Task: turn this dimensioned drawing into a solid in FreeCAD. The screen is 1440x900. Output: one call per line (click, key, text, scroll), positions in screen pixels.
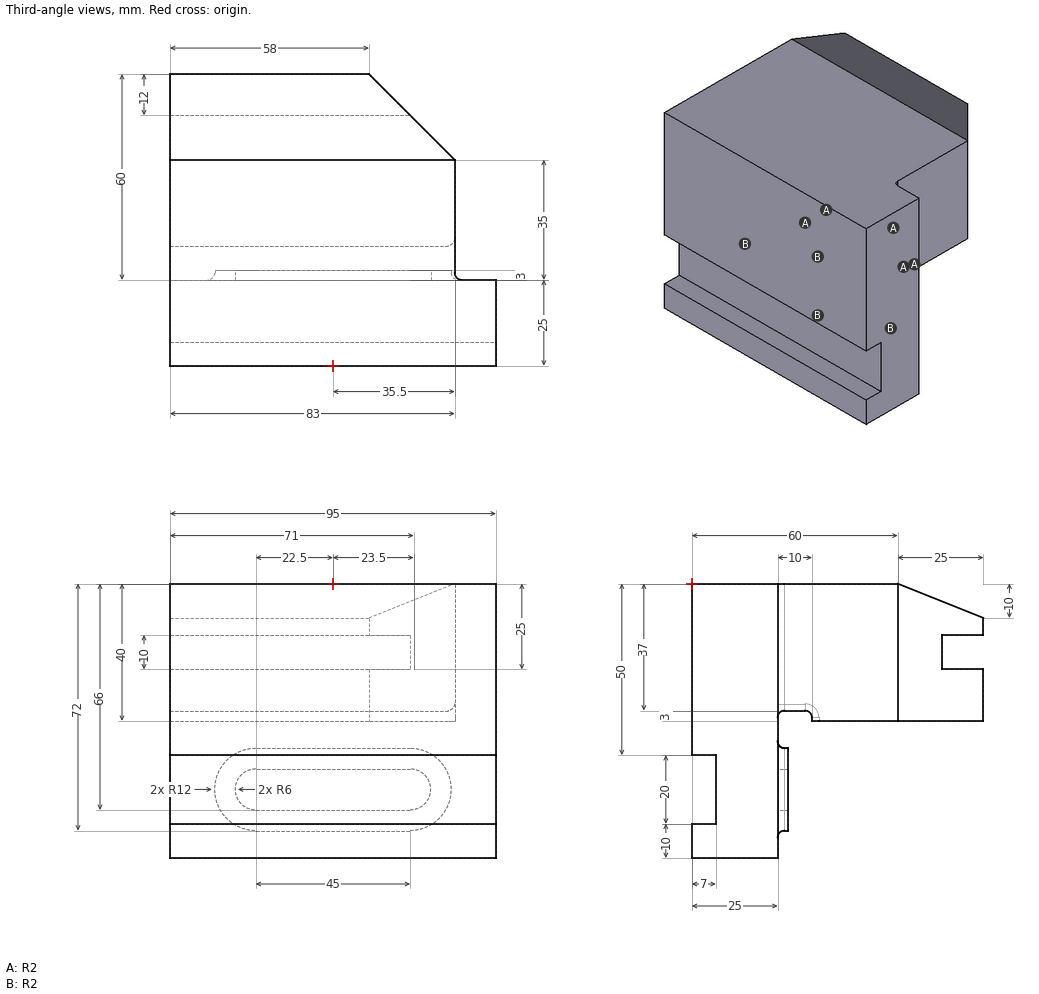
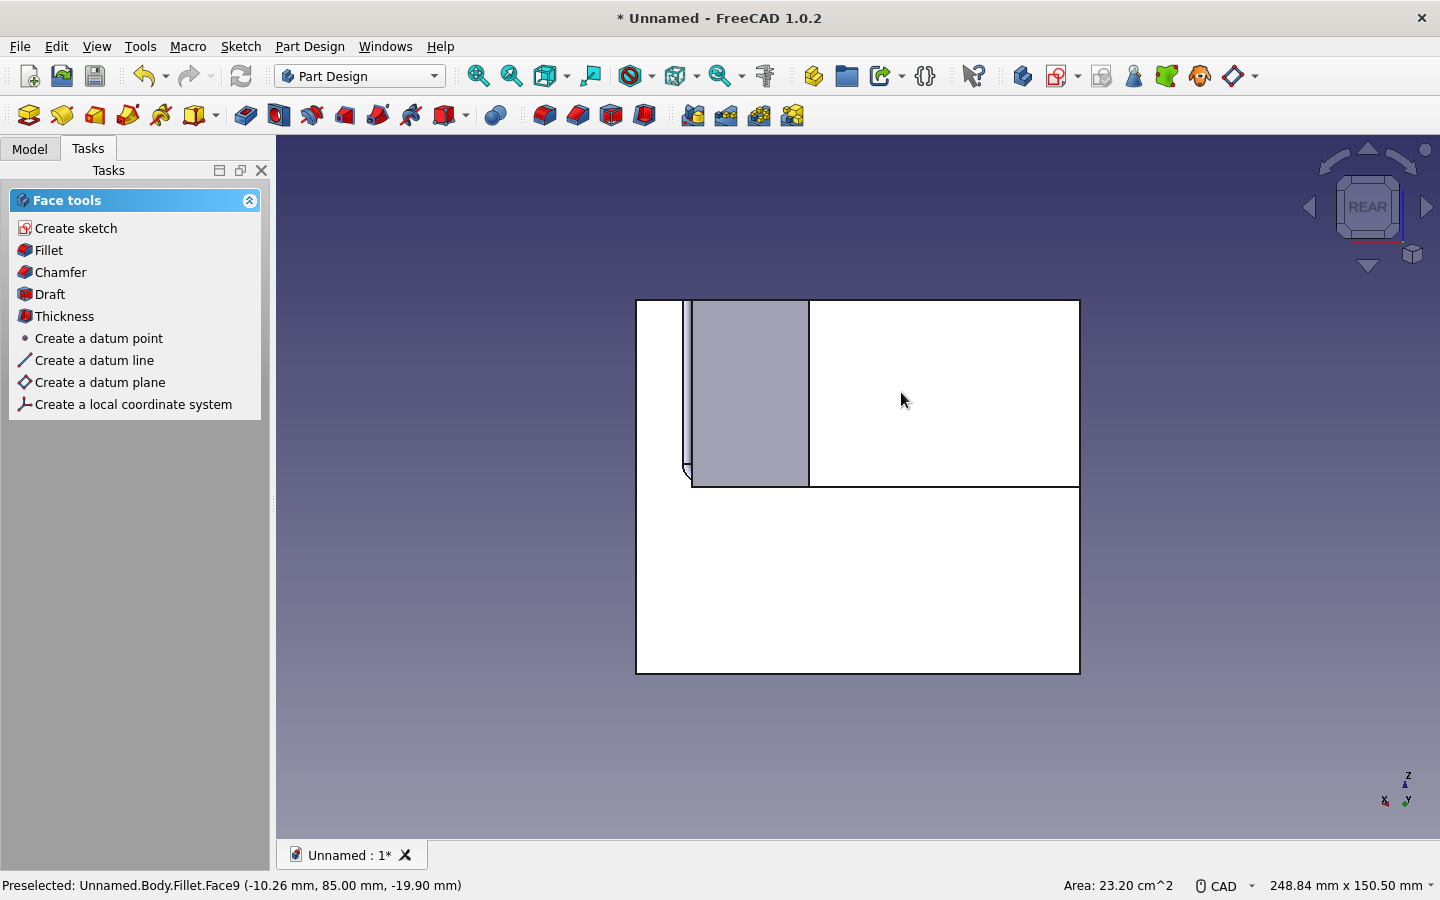
click(1056, 76)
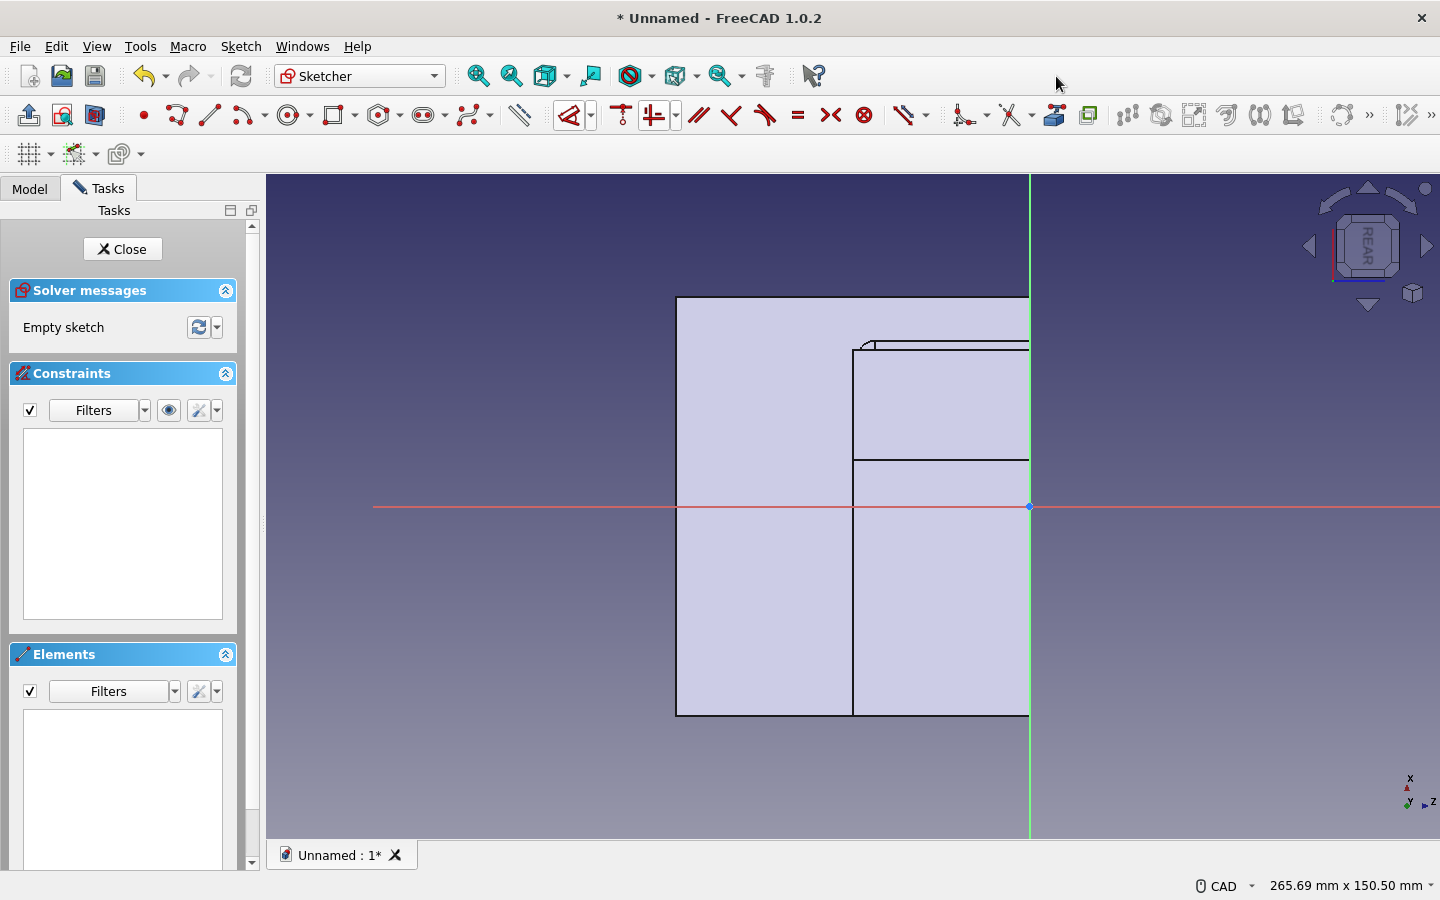
scroll(1275, 667, up, 2)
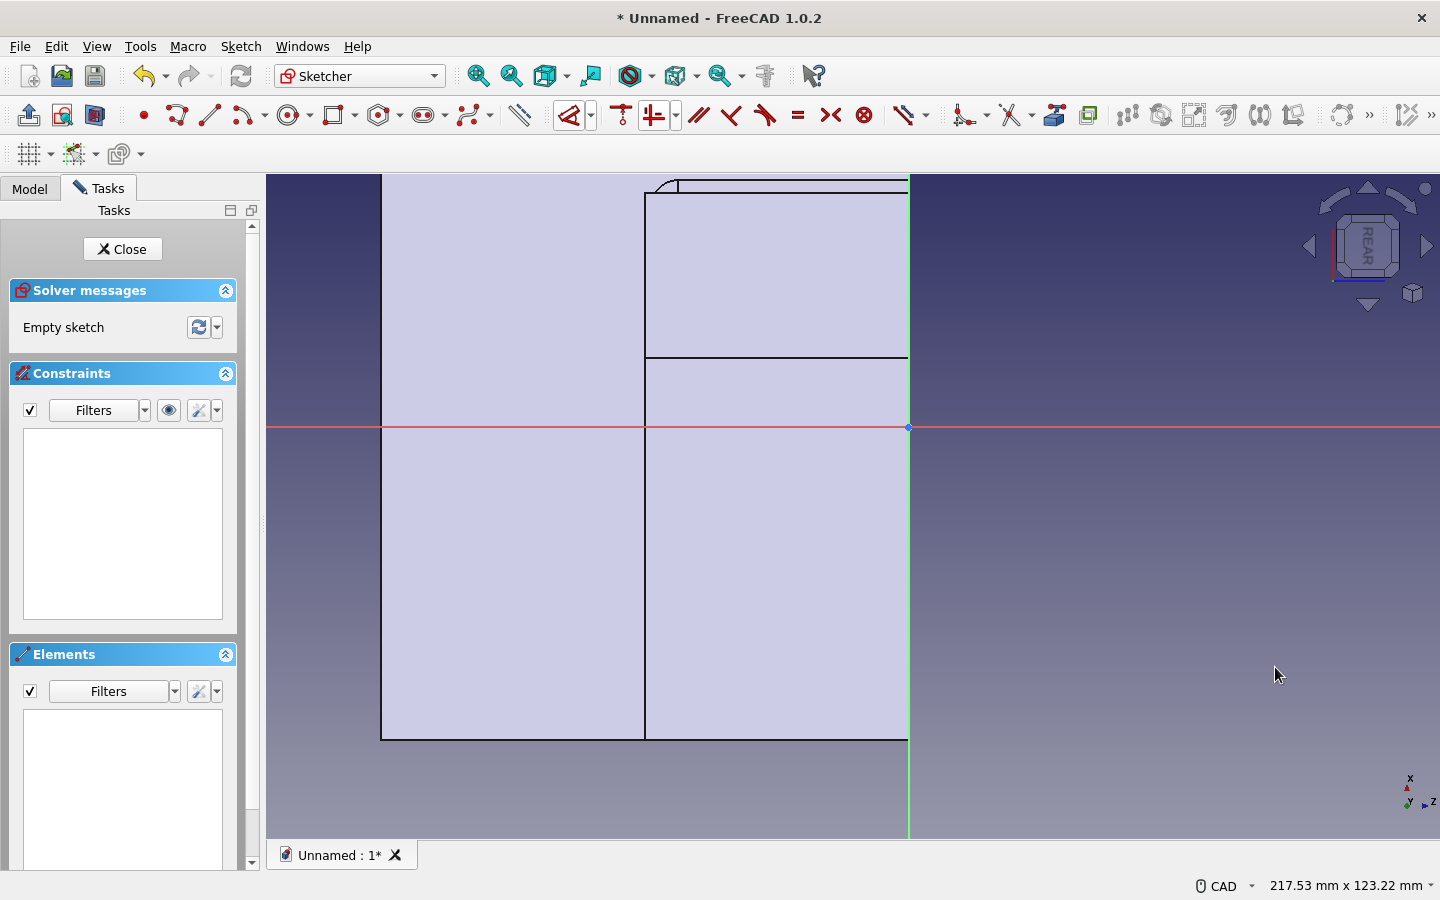
click(332, 116)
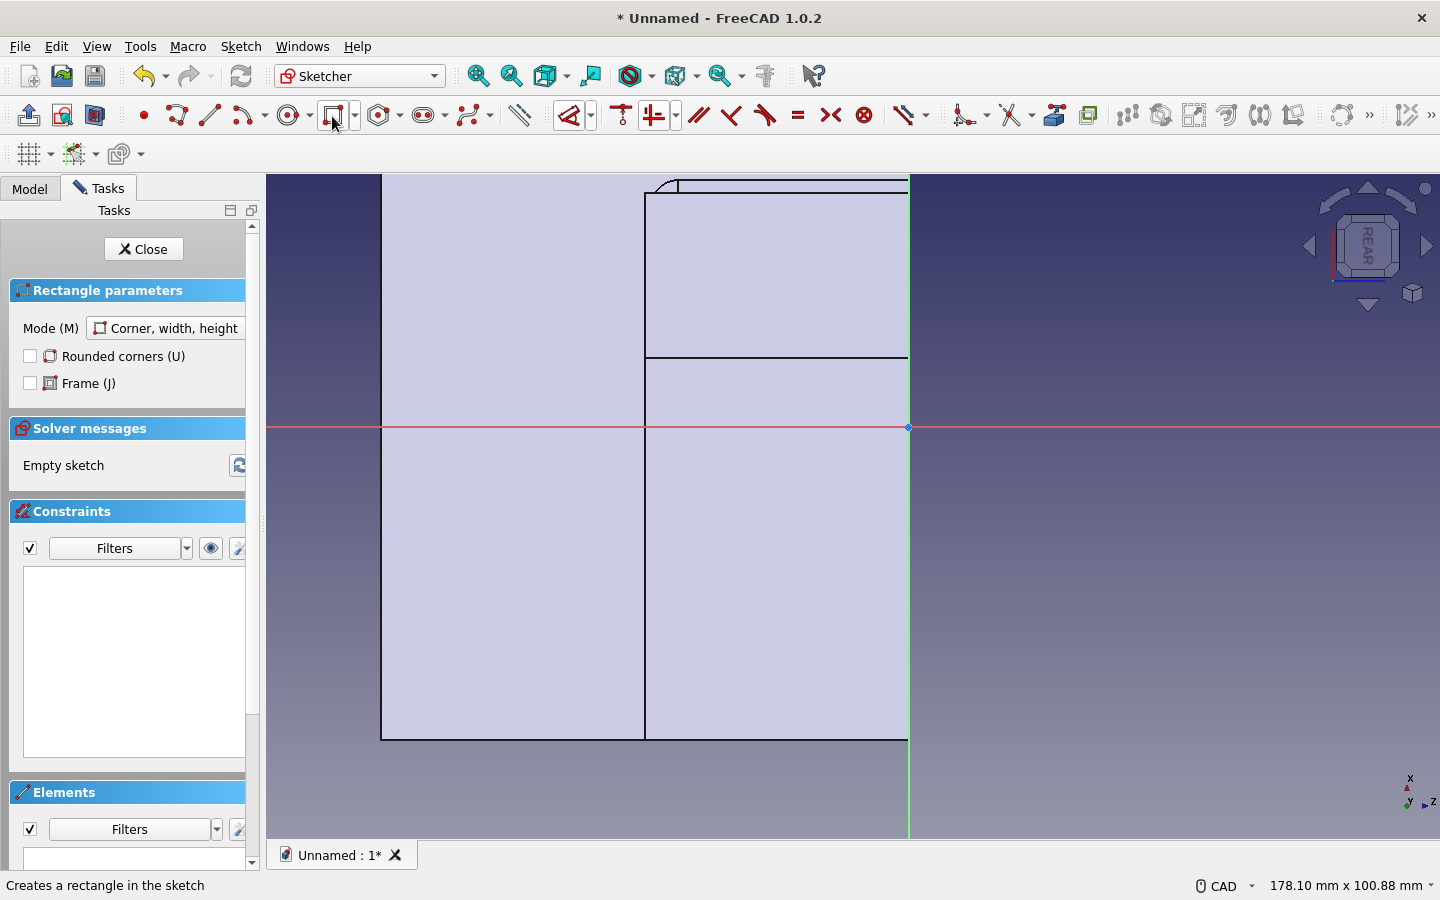
click(744, 272)
click(810, 740)
key(Escape)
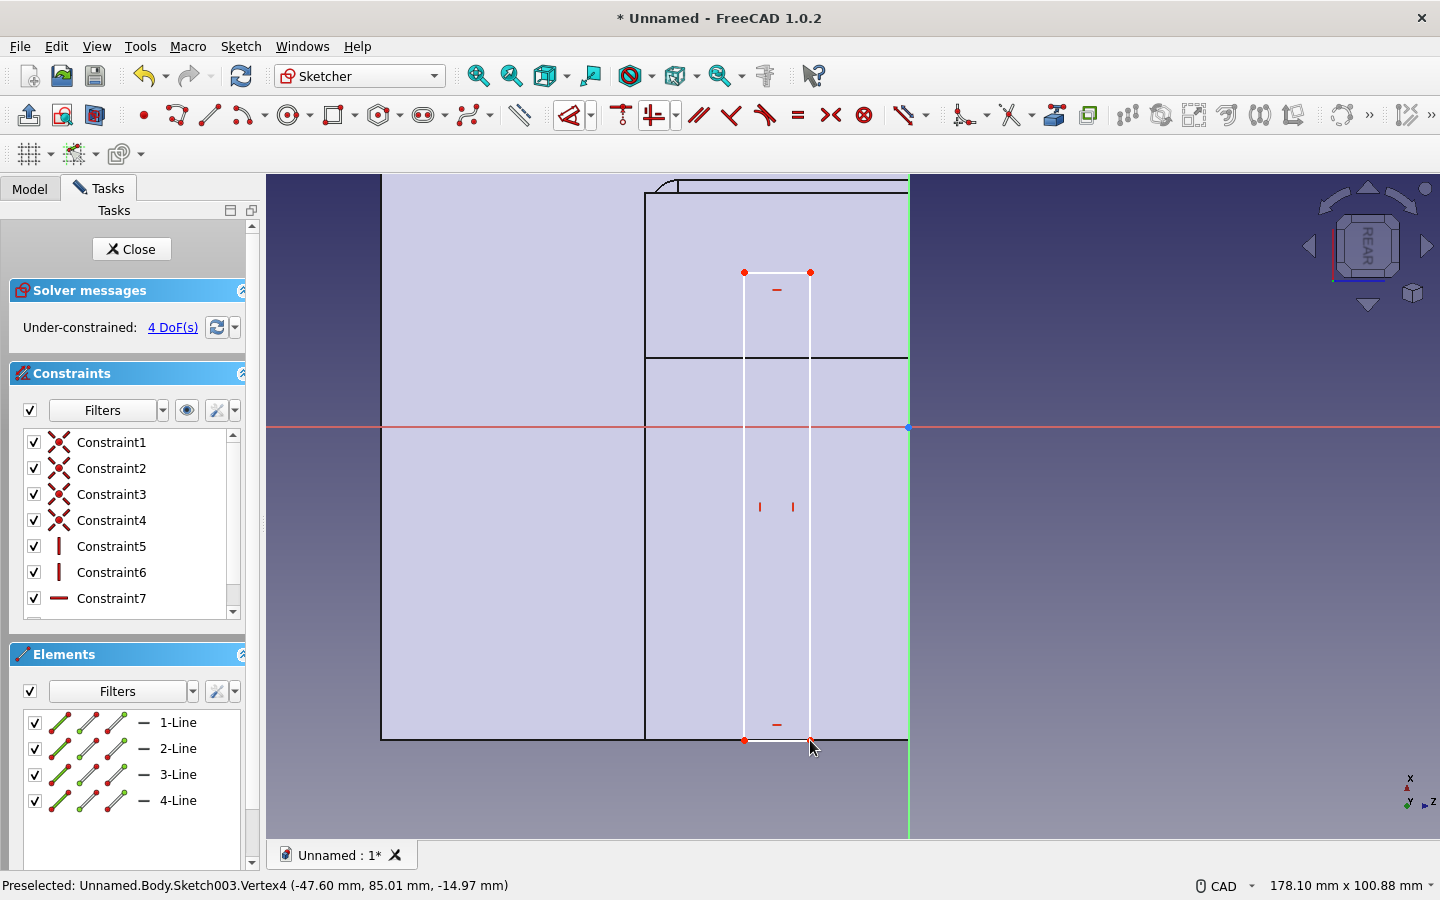
click(744, 413)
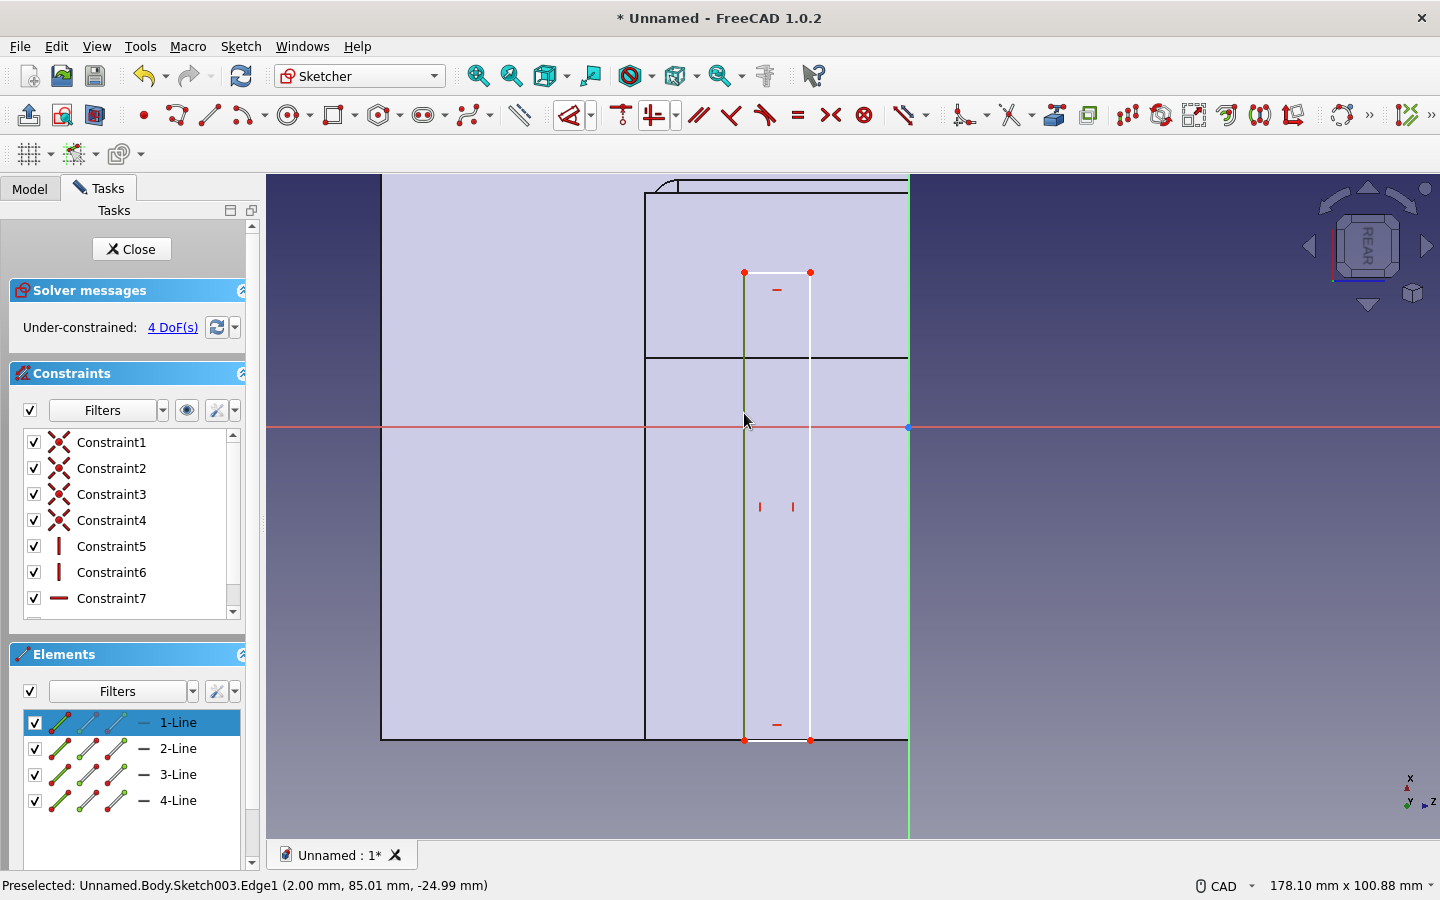
key(i)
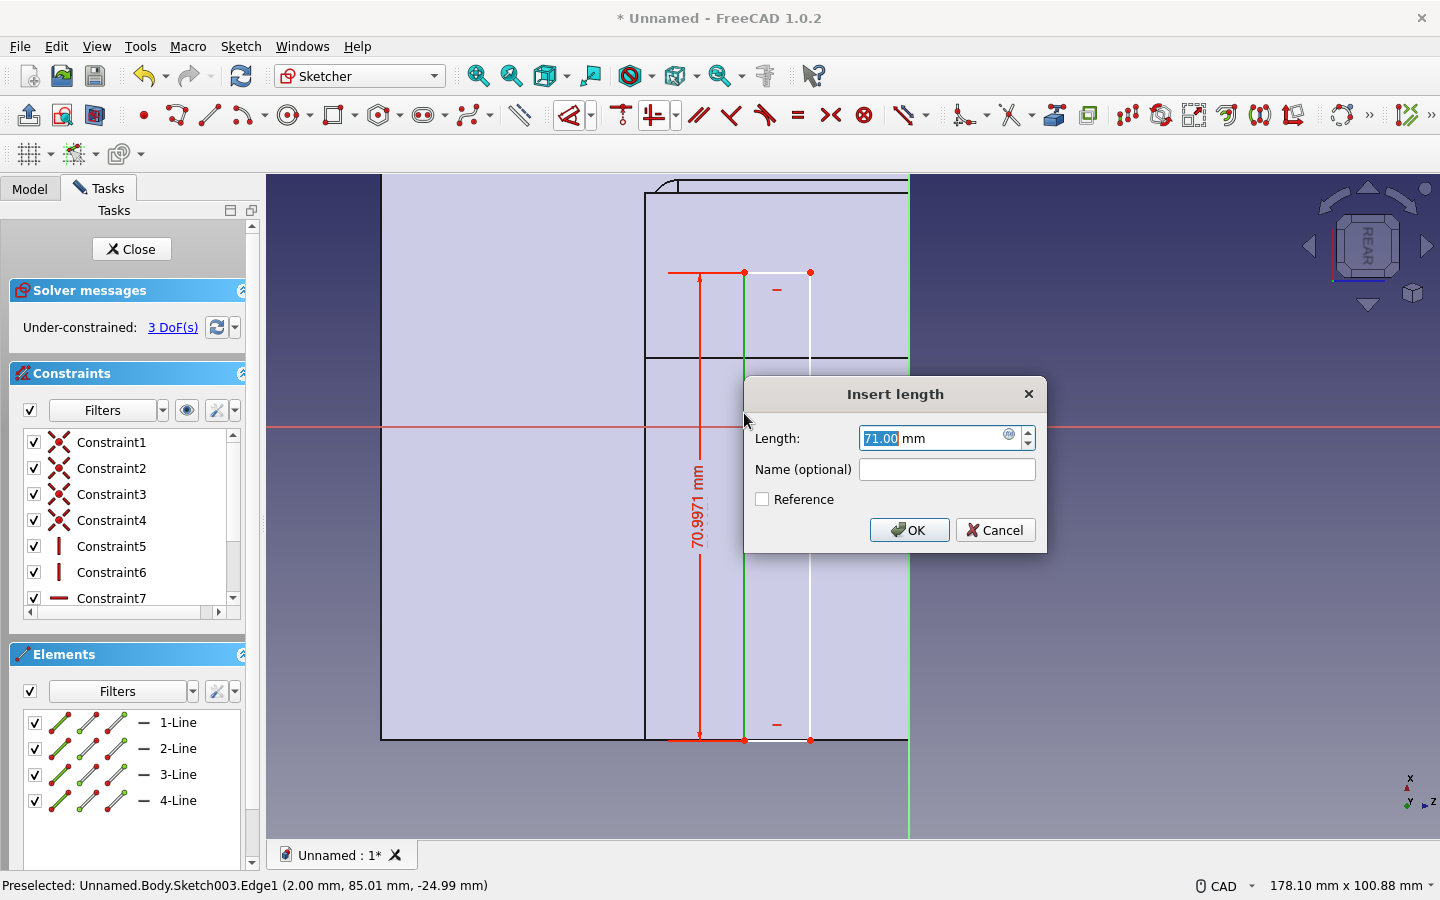
text(71)
key(Return)